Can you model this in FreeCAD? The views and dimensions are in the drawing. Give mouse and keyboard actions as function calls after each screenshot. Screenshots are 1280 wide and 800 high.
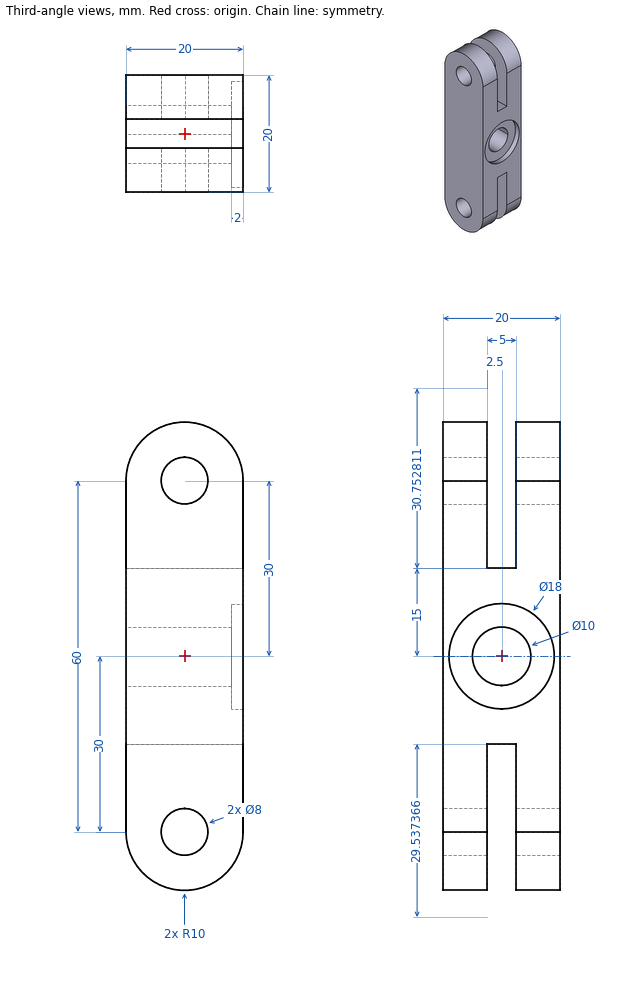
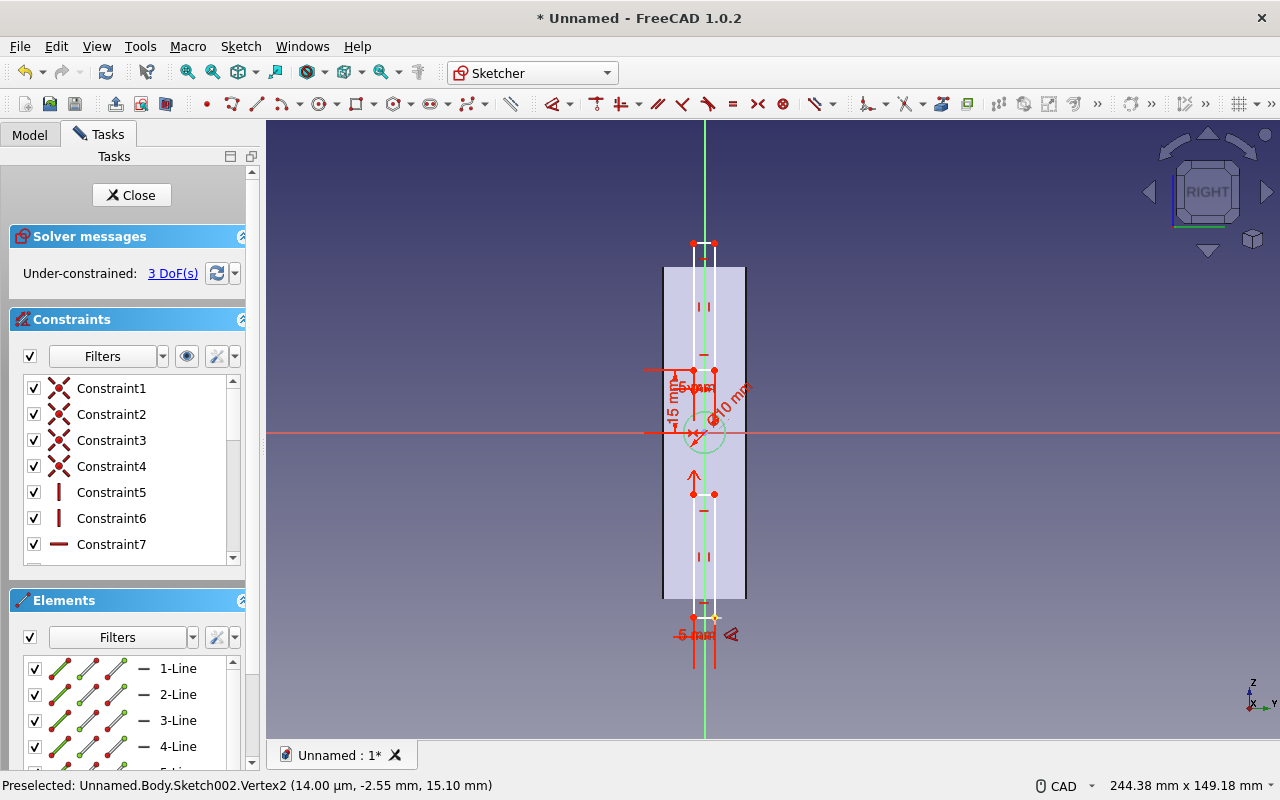
scroll(694, 243, up, 7)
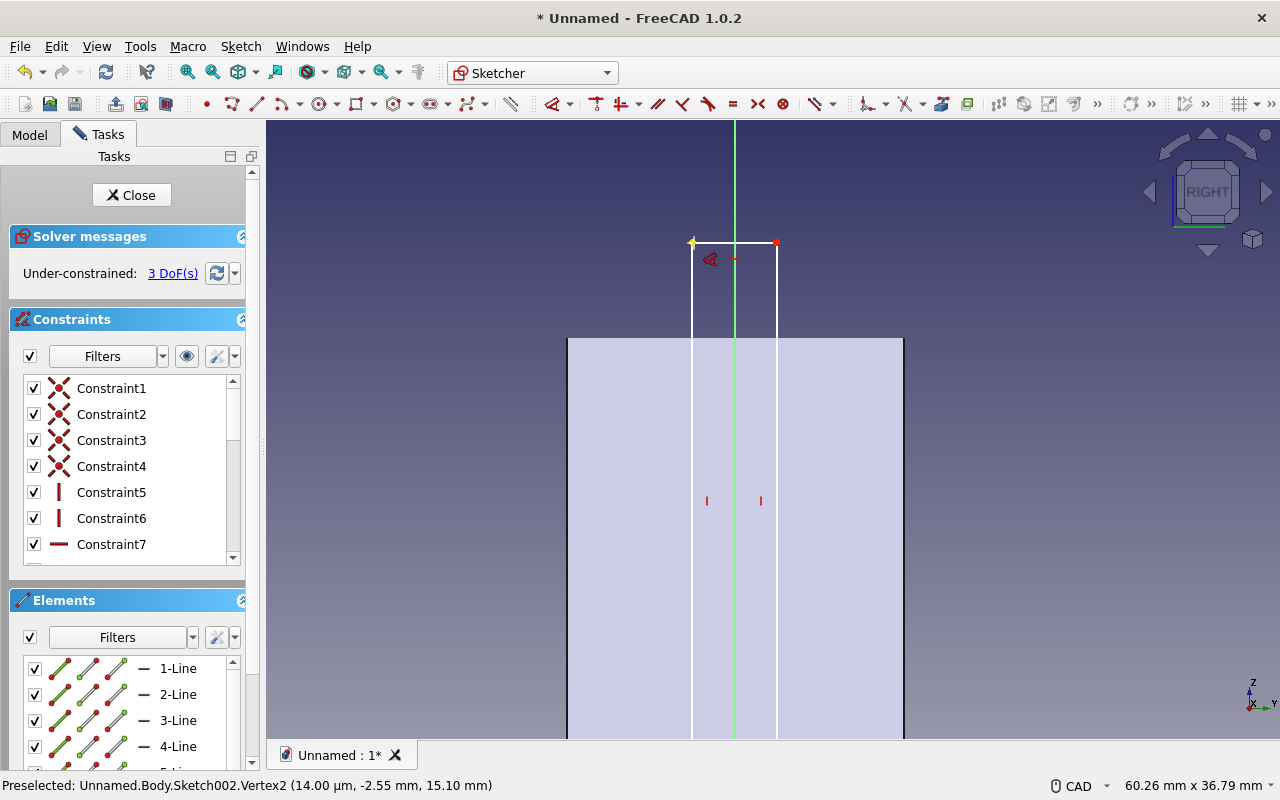
click(692, 243)
click(714, 209)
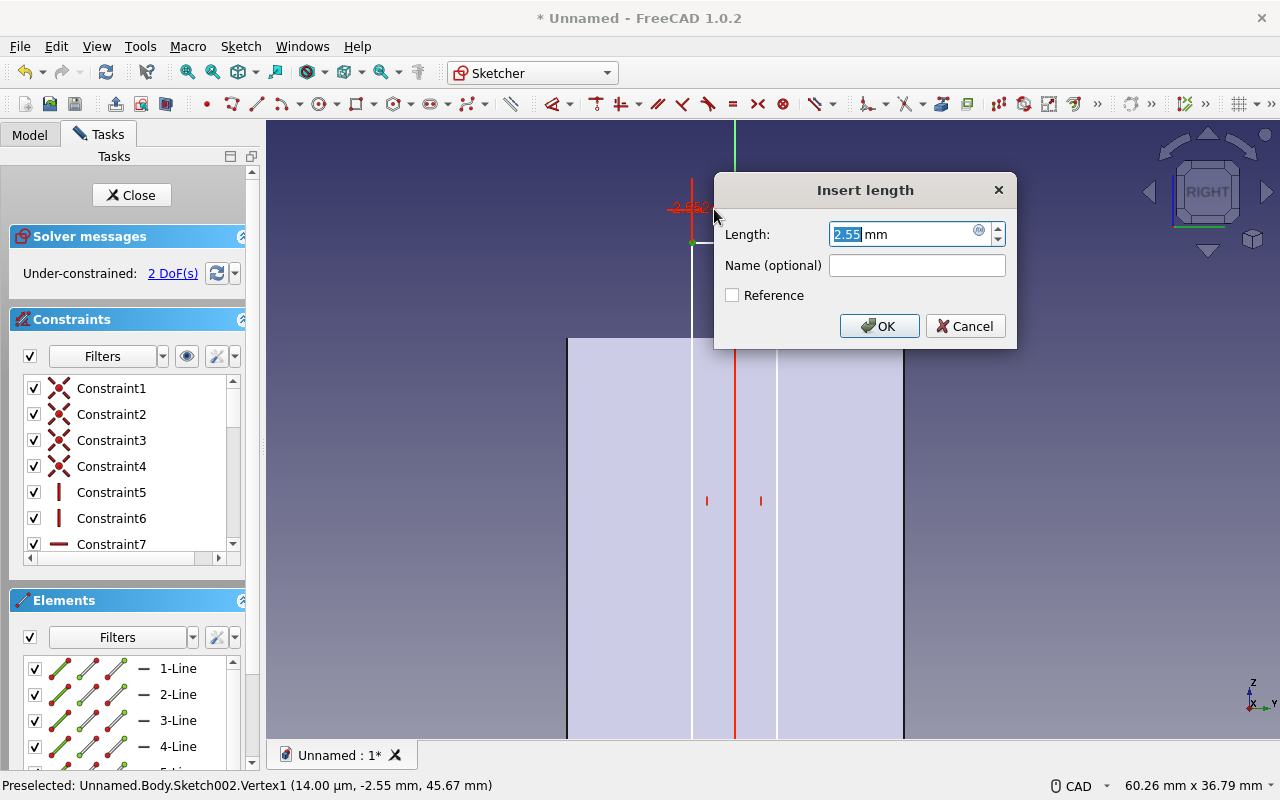
text(2.5)
key(Return)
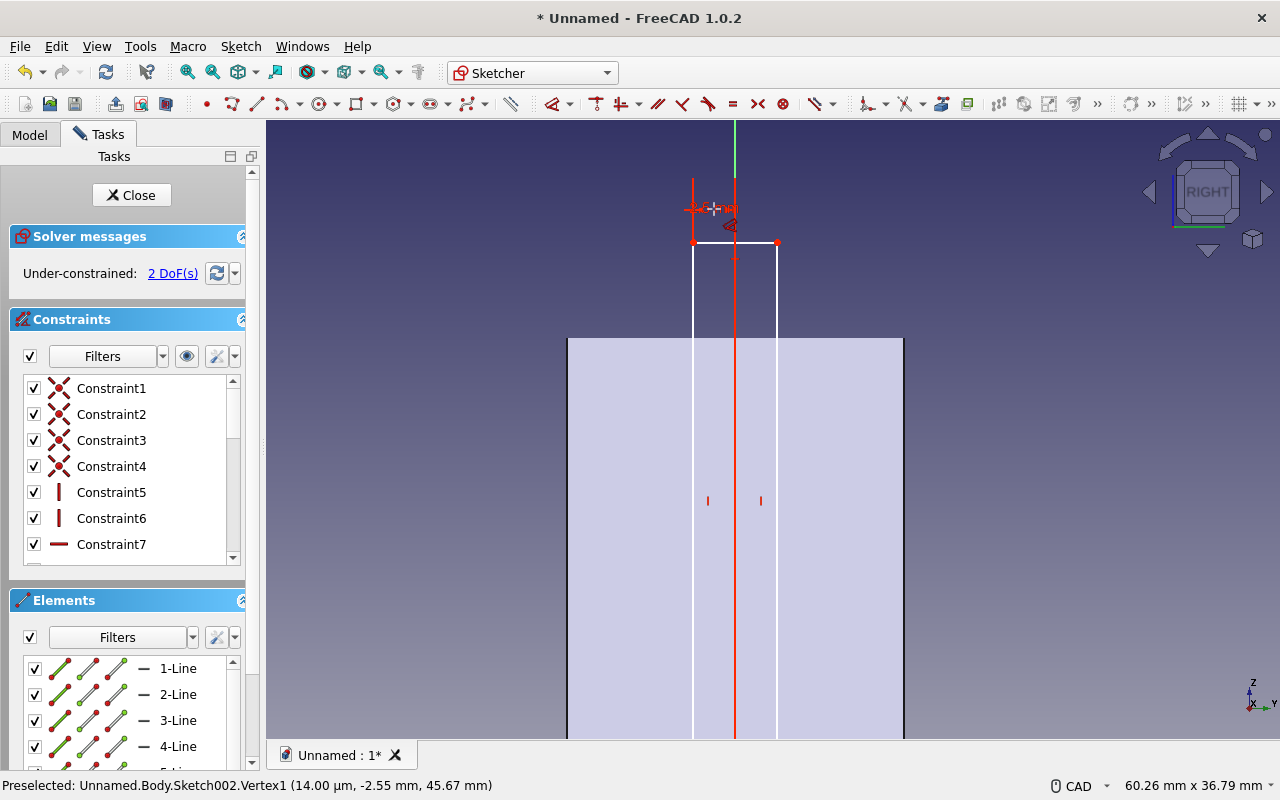
scroll(694, 242, down, 7)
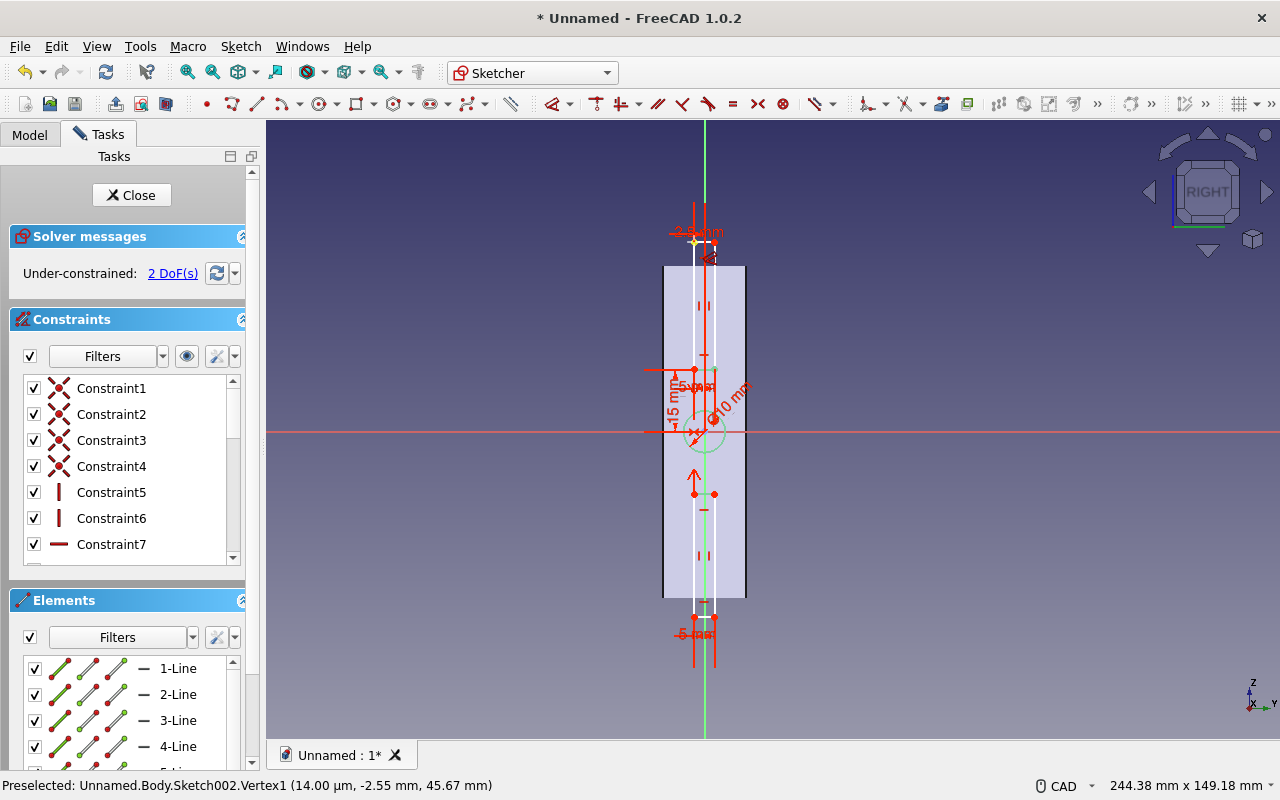
scroll(694, 281, up, 2)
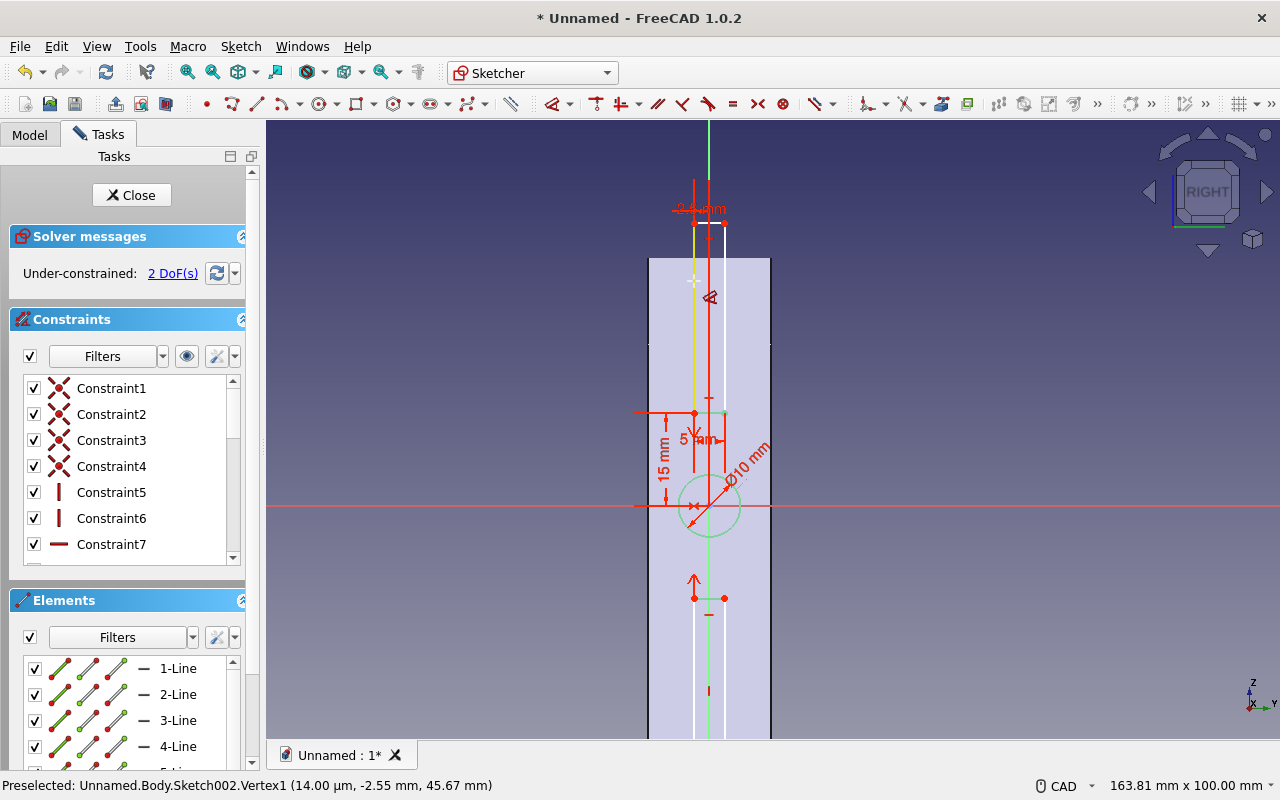
click(694, 280)
click(660, 318)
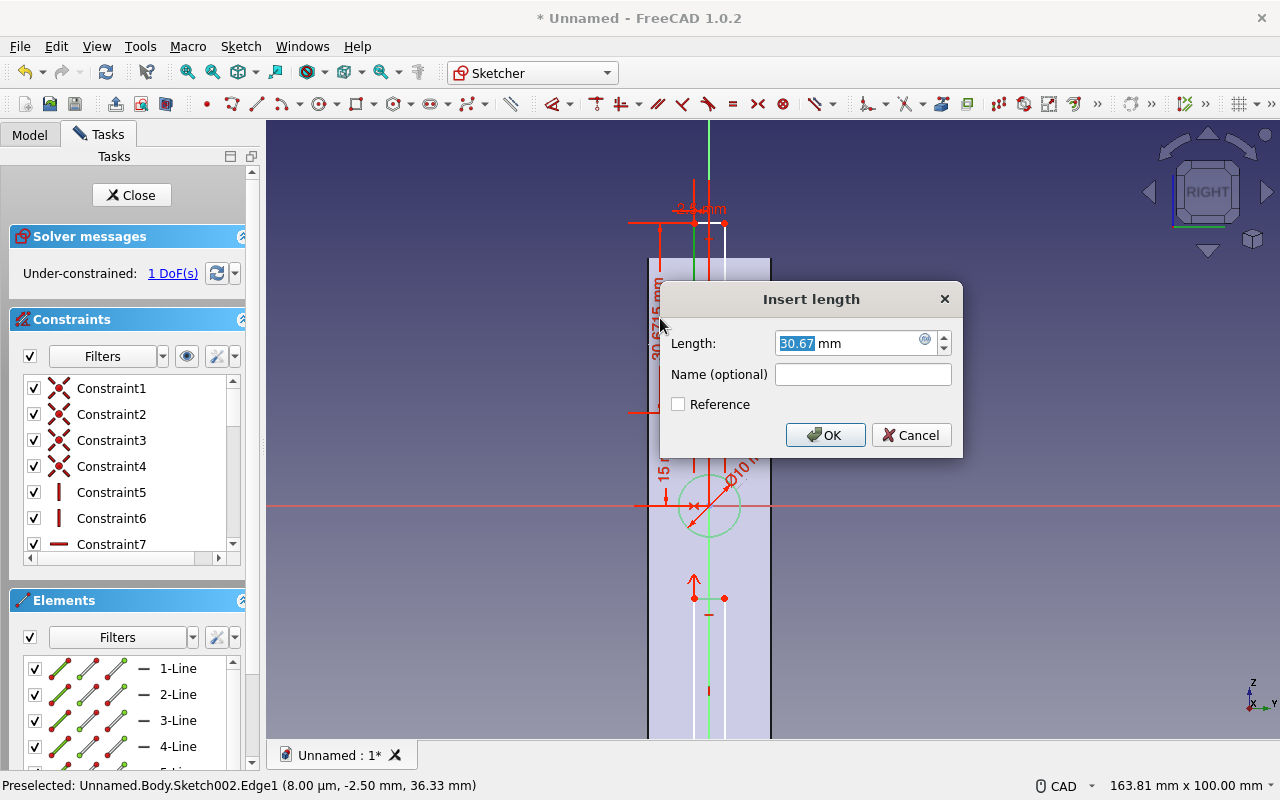
text(30.752811)
key(Return)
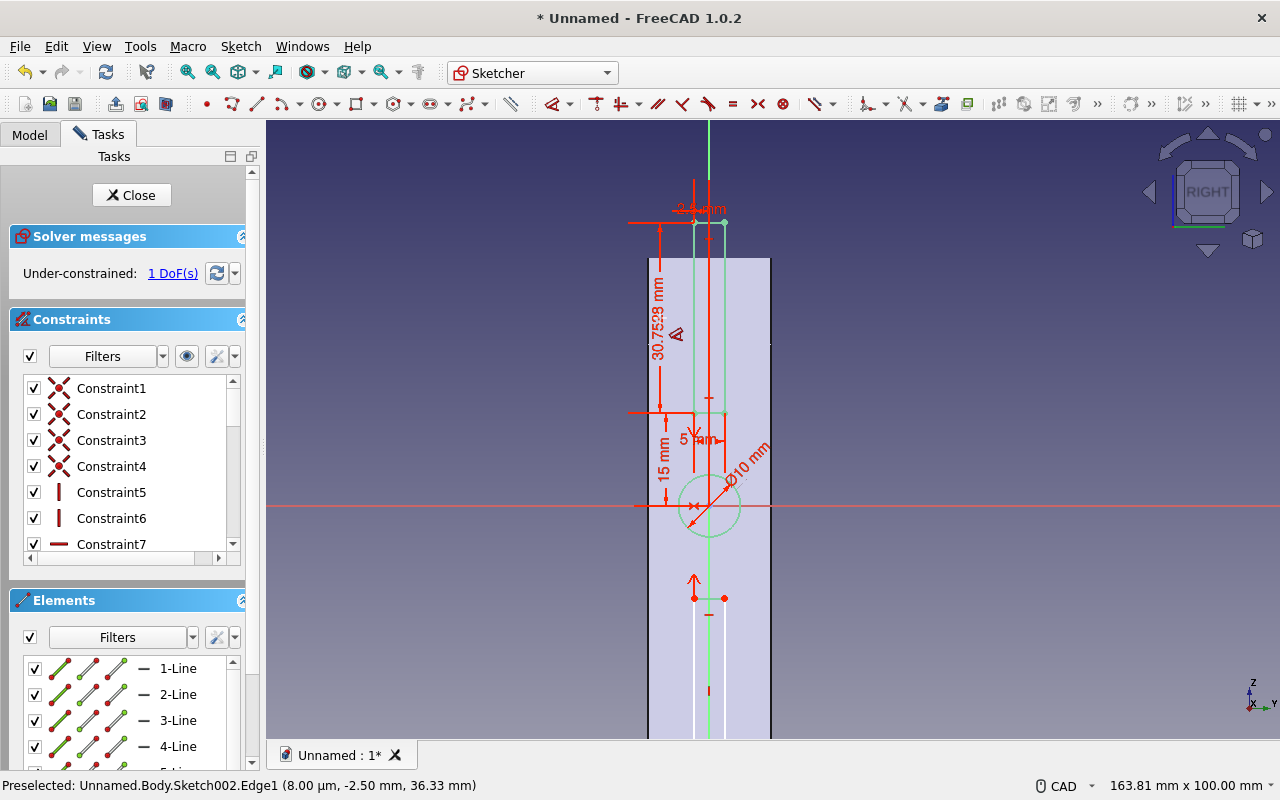
click(694, 654)
click(660, 655)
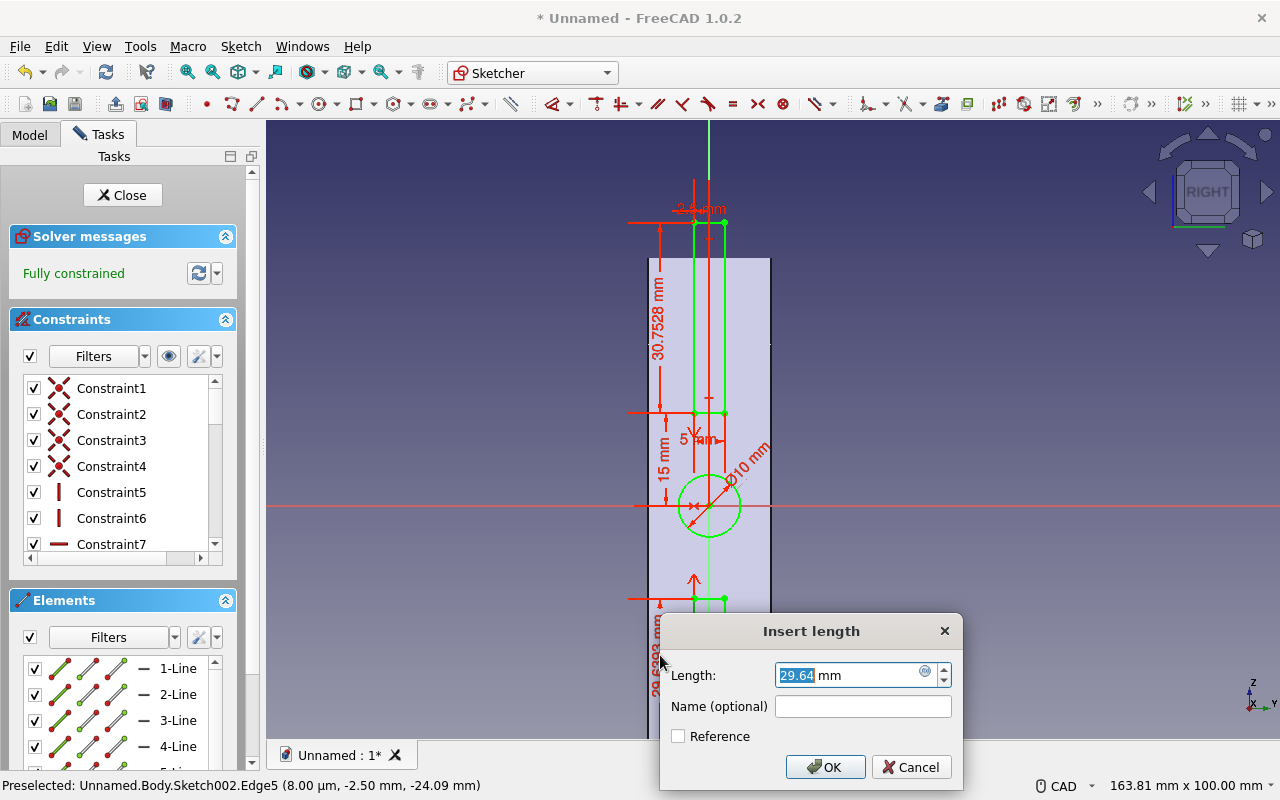
text(29.537366)
key(Return)
key(Escape)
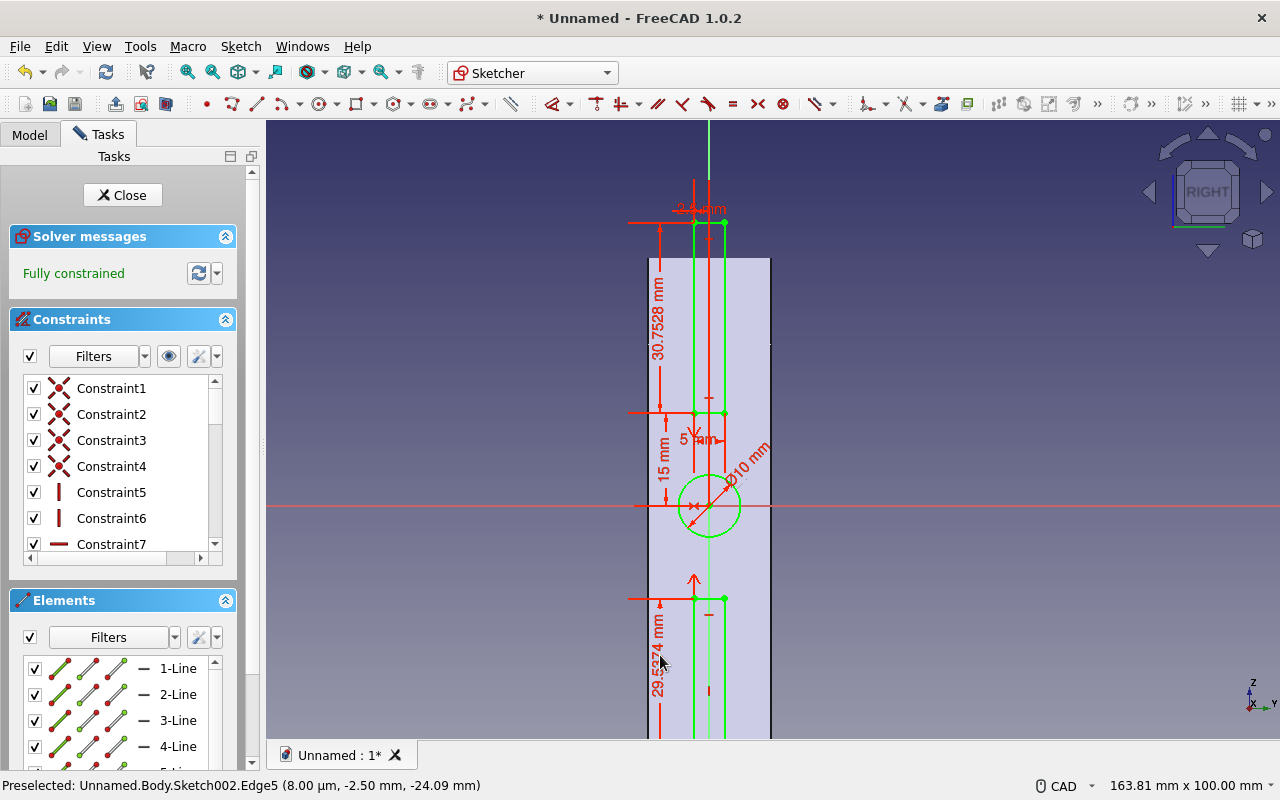
click(123, 195)